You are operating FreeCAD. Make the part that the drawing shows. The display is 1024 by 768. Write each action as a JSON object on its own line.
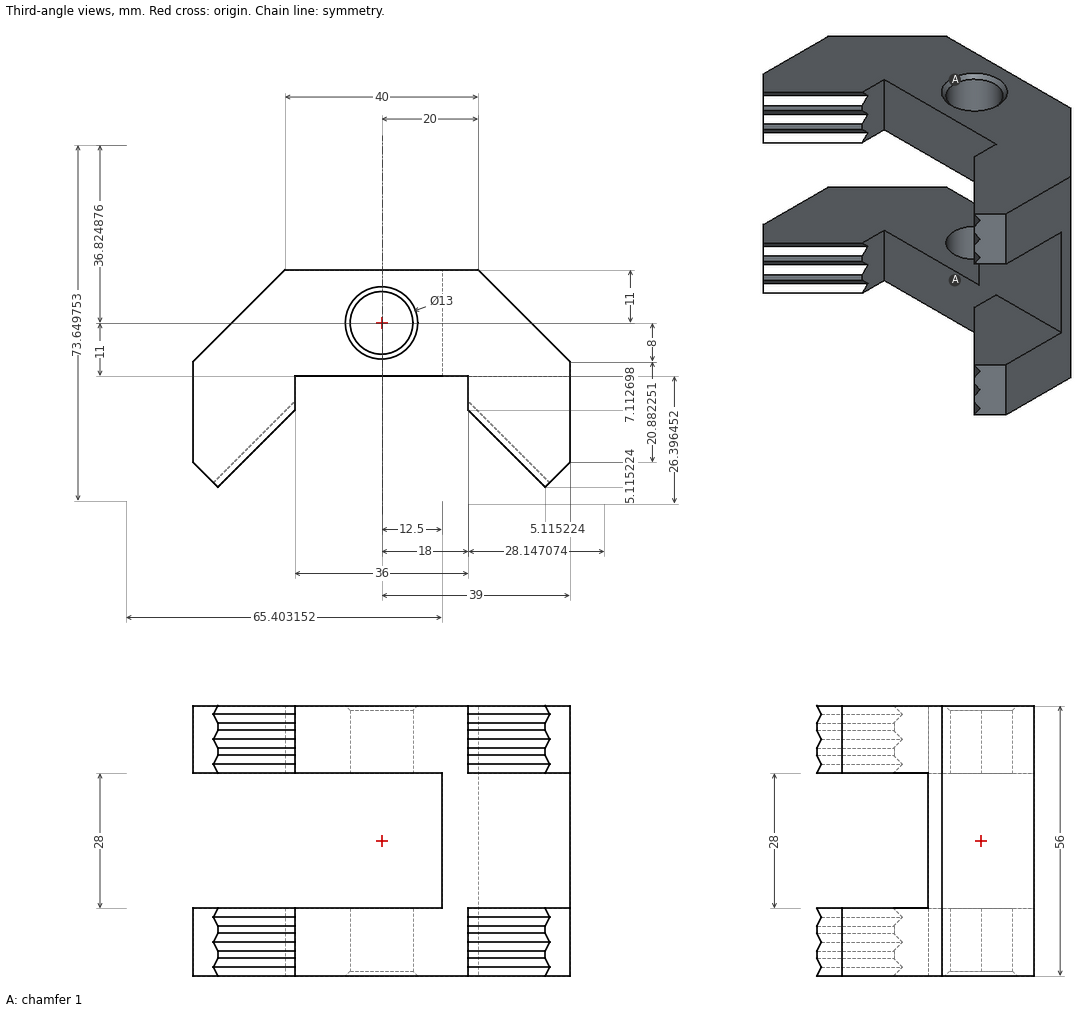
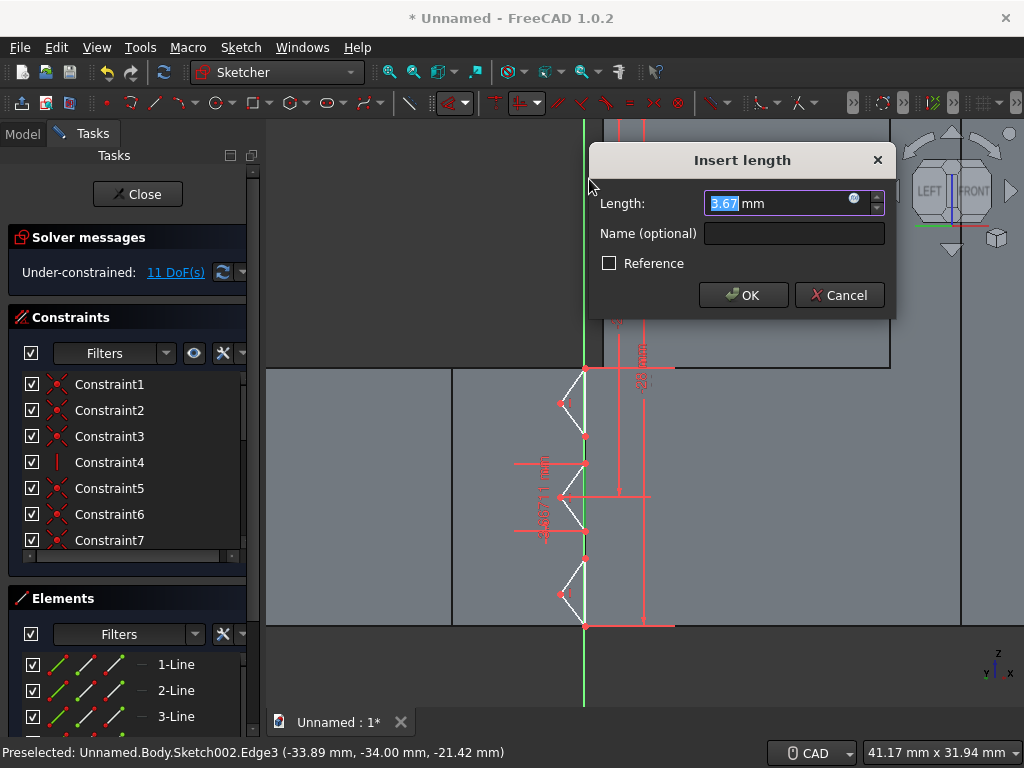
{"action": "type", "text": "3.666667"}
{"action": "key", "text": "Return"}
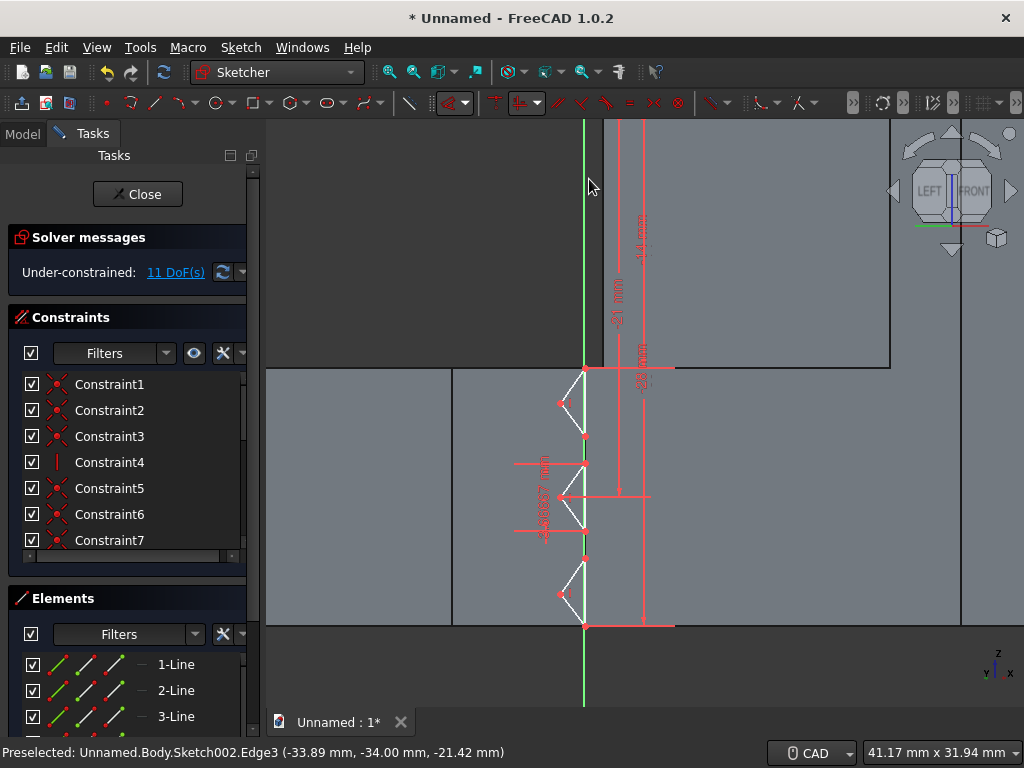
{"action": "left_click", "coordinate": [585, 416]}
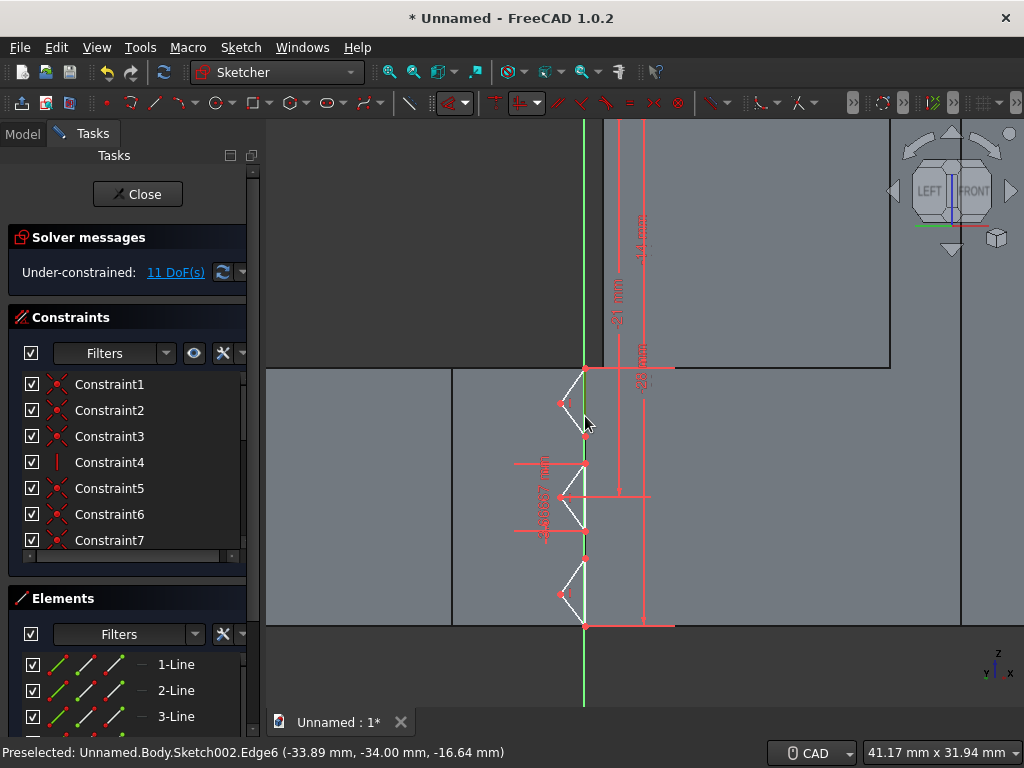
{"action": "left_click", "coordinate": [468, 104]}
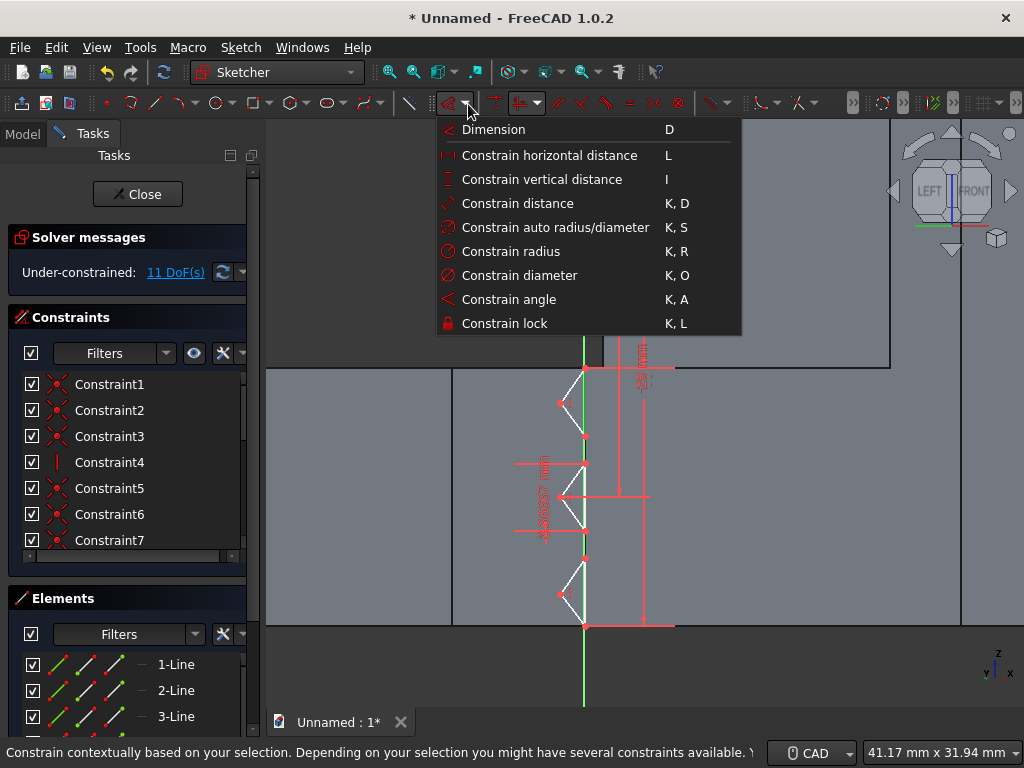
{"action": "left_click", "coordinate": [589, 179]}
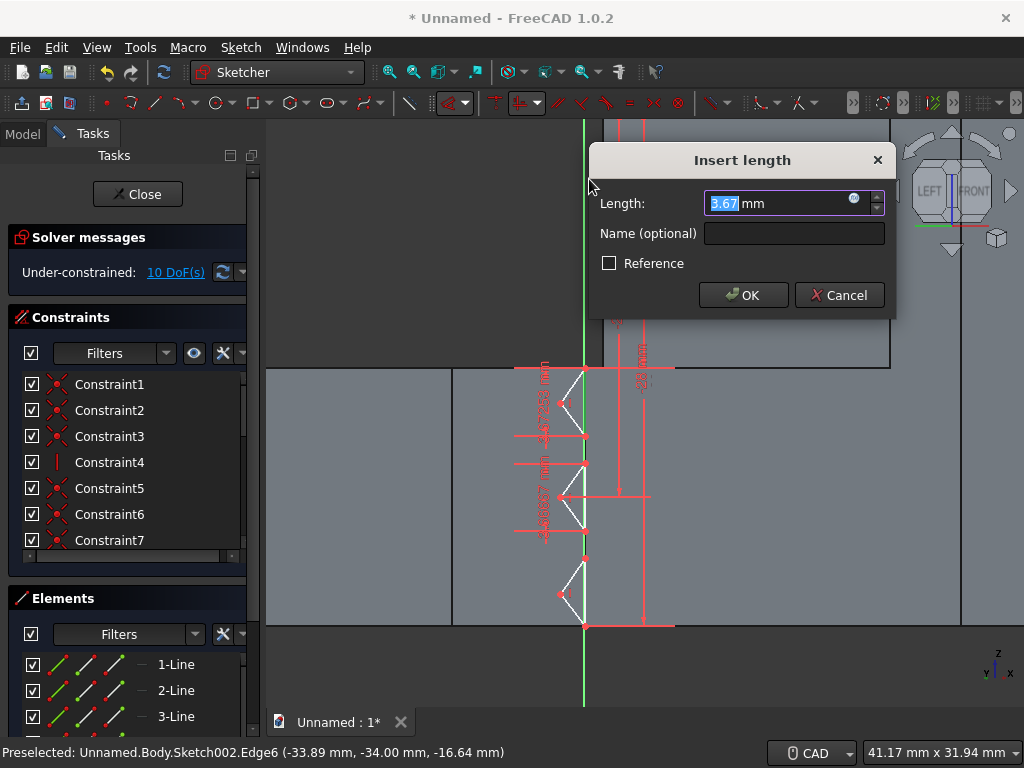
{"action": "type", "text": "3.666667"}
{"action": "key", "text": "Return"}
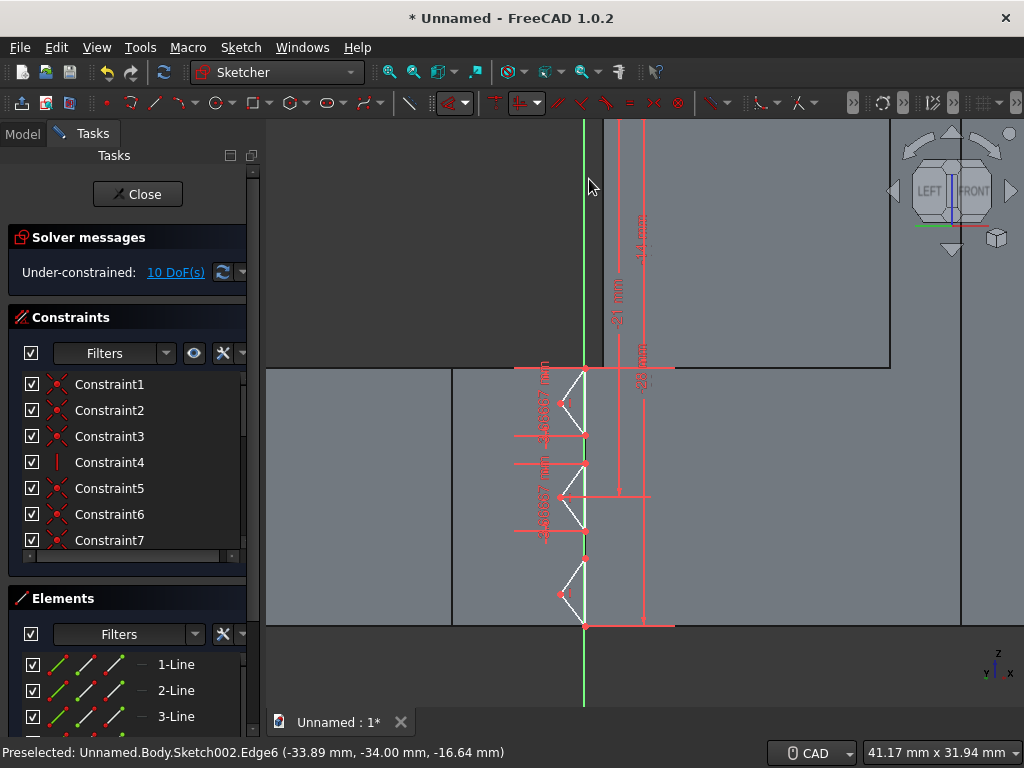
{"action": "left_click", "coordinate": [585, 606]}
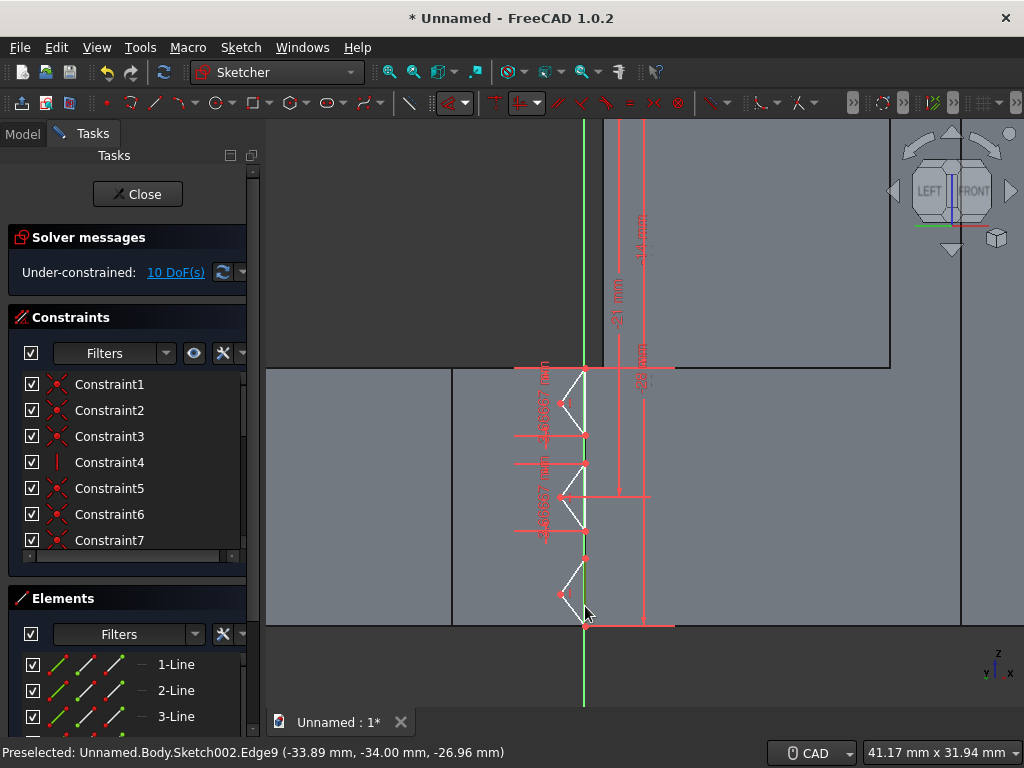
{"action": "key", "text": "i"}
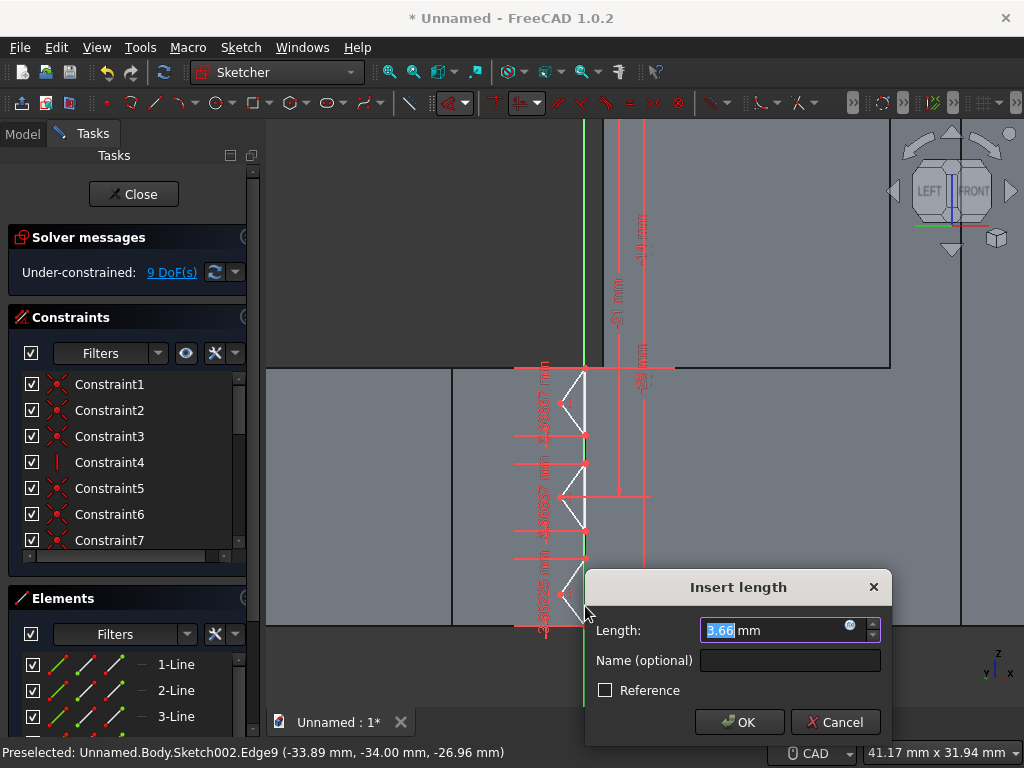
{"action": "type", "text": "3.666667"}
{"action": "key", "text": "Return"}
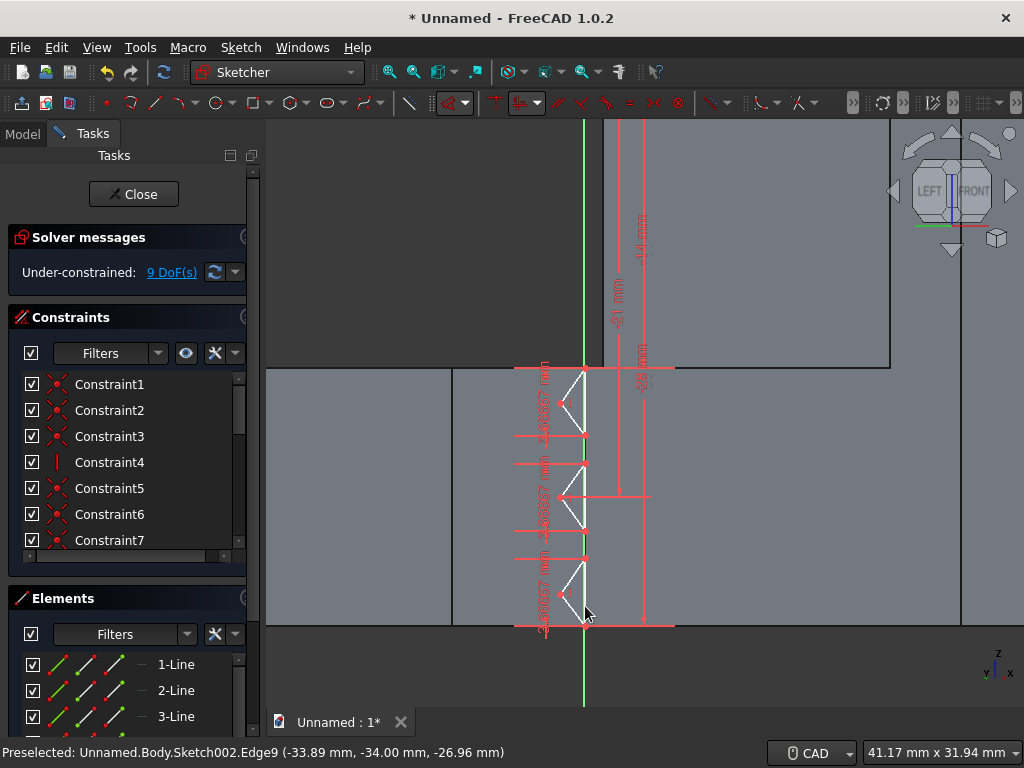
{"action": "scroll", "coordinate": [585, 464], "scroll_direction": "up", "scroll_amount": 17}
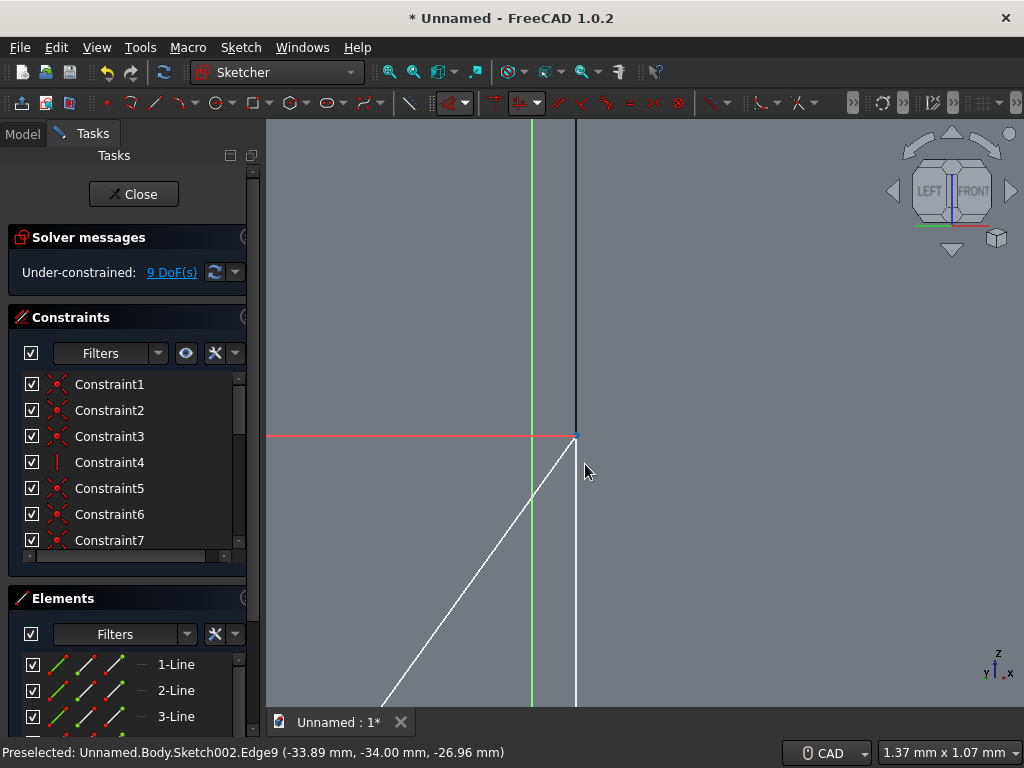
{"action": "left_click", "coordinate": [576, 436]}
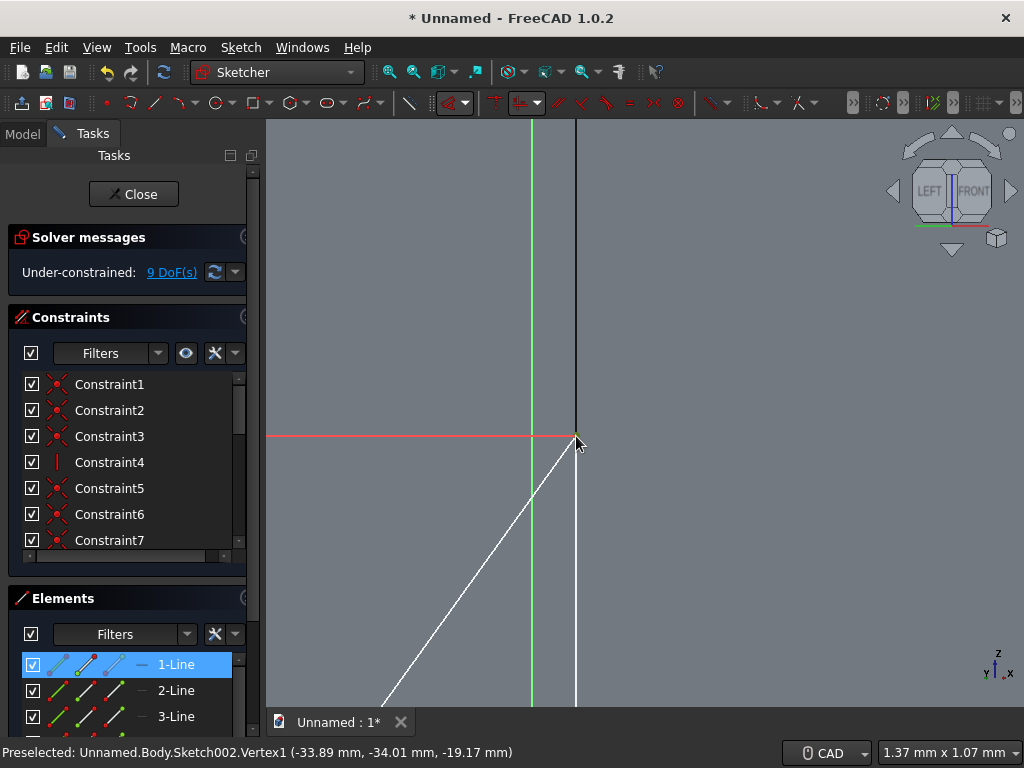
{"action": "left_click", "coordinate": [468, 104]}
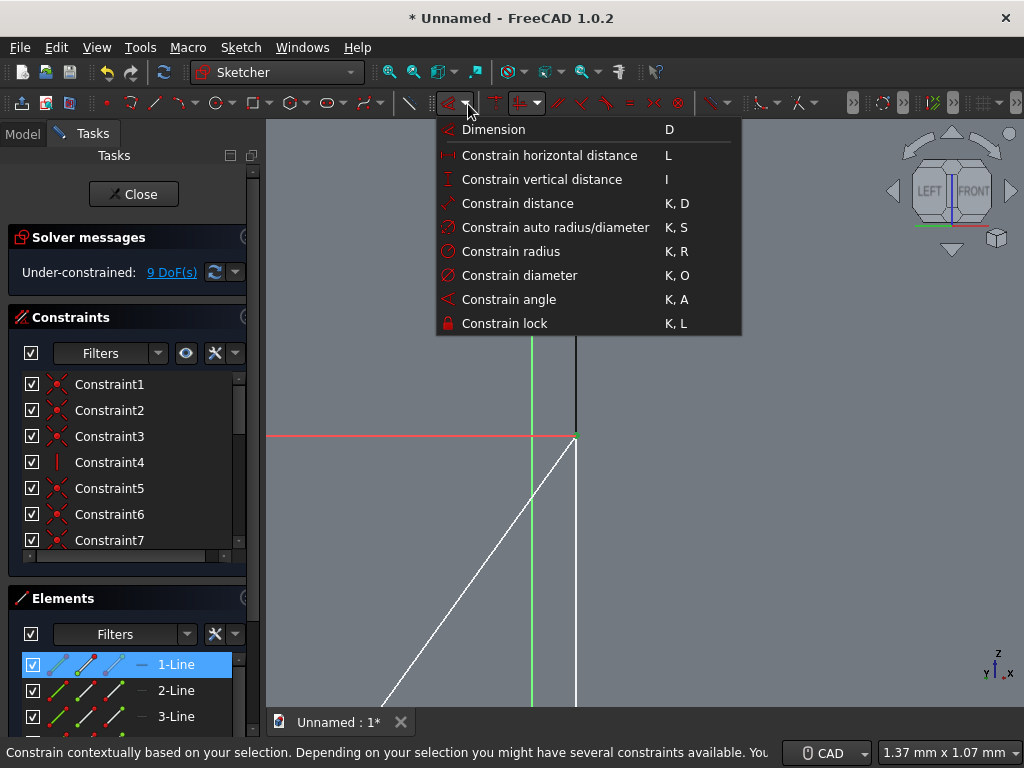
{"action": "left_click", "coordinate": [589, 155]}